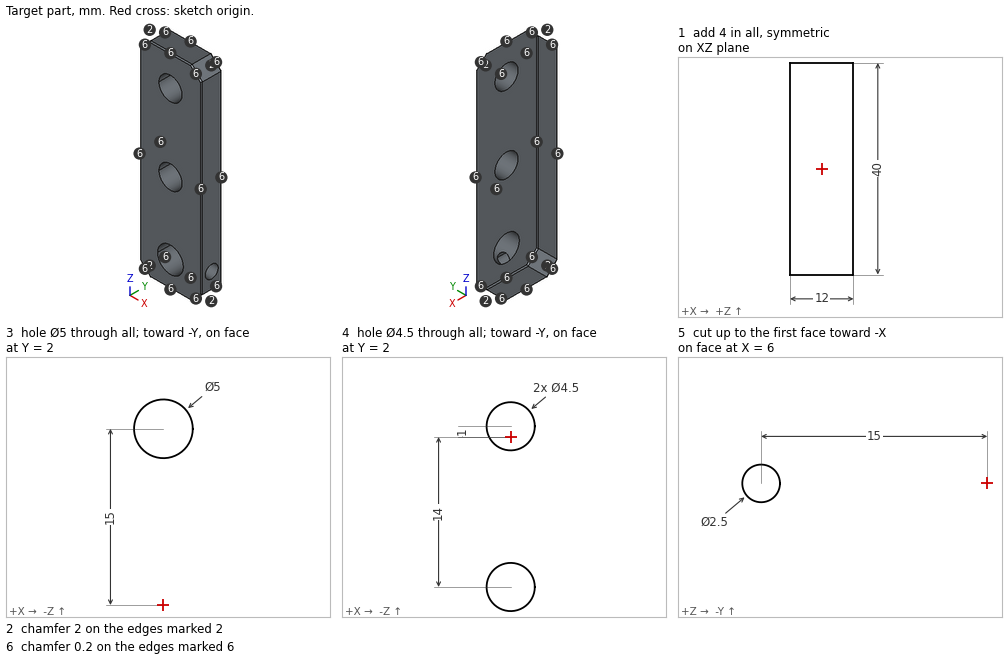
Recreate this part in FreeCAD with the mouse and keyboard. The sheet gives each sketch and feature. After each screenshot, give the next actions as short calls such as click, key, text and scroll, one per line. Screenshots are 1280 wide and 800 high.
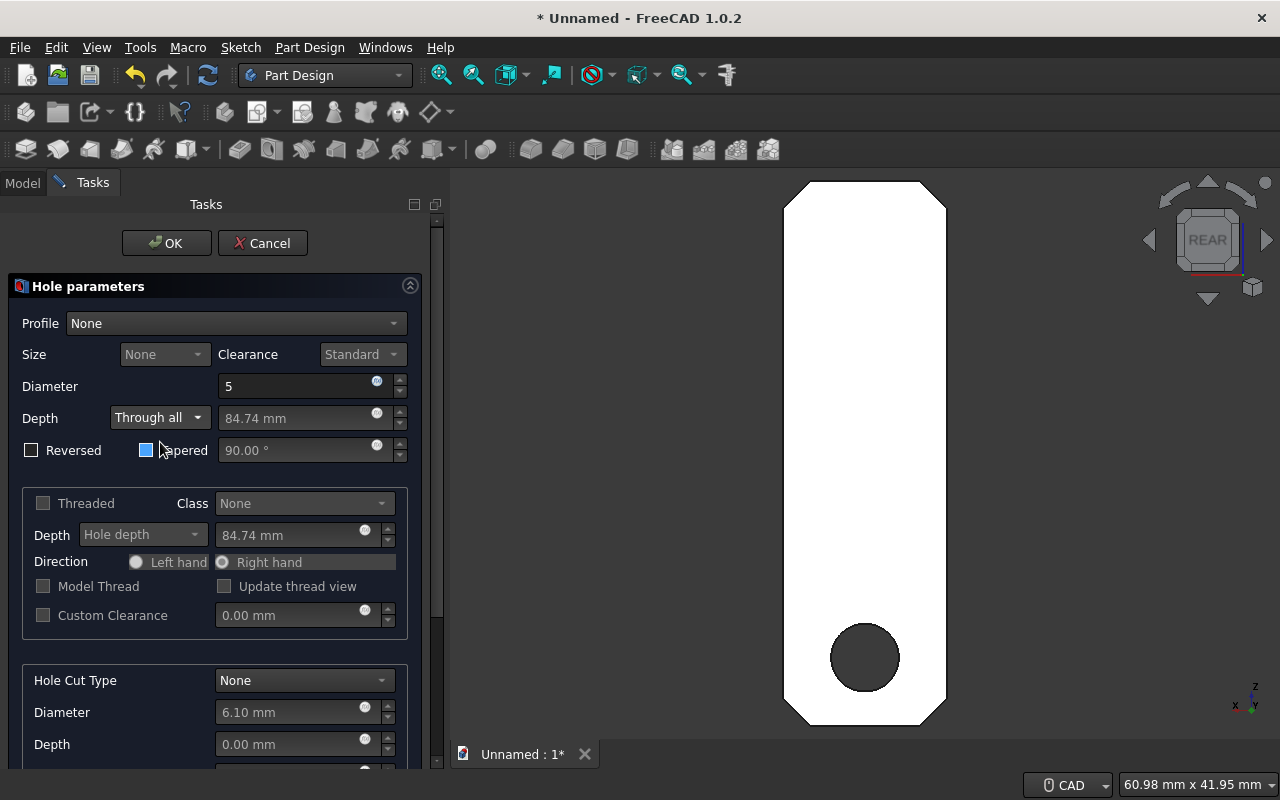
click(167, 243)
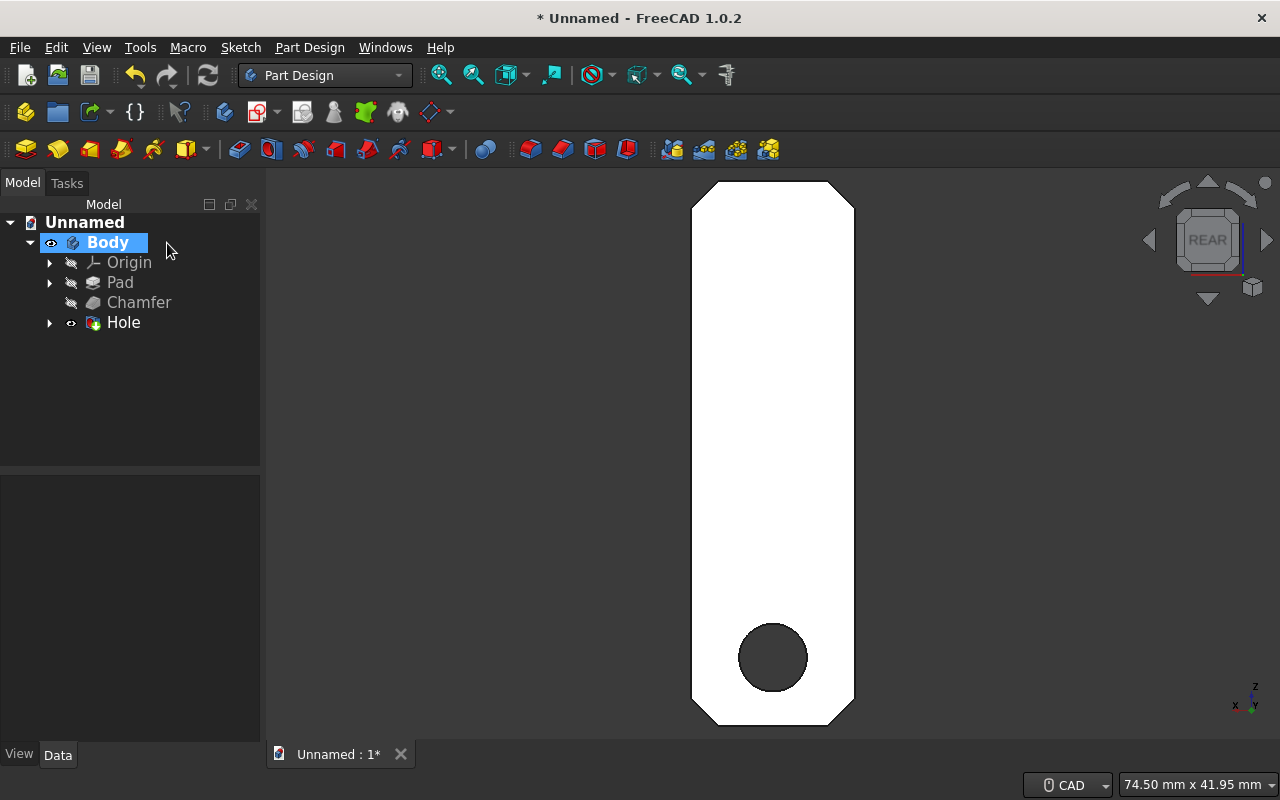
click(773, 297)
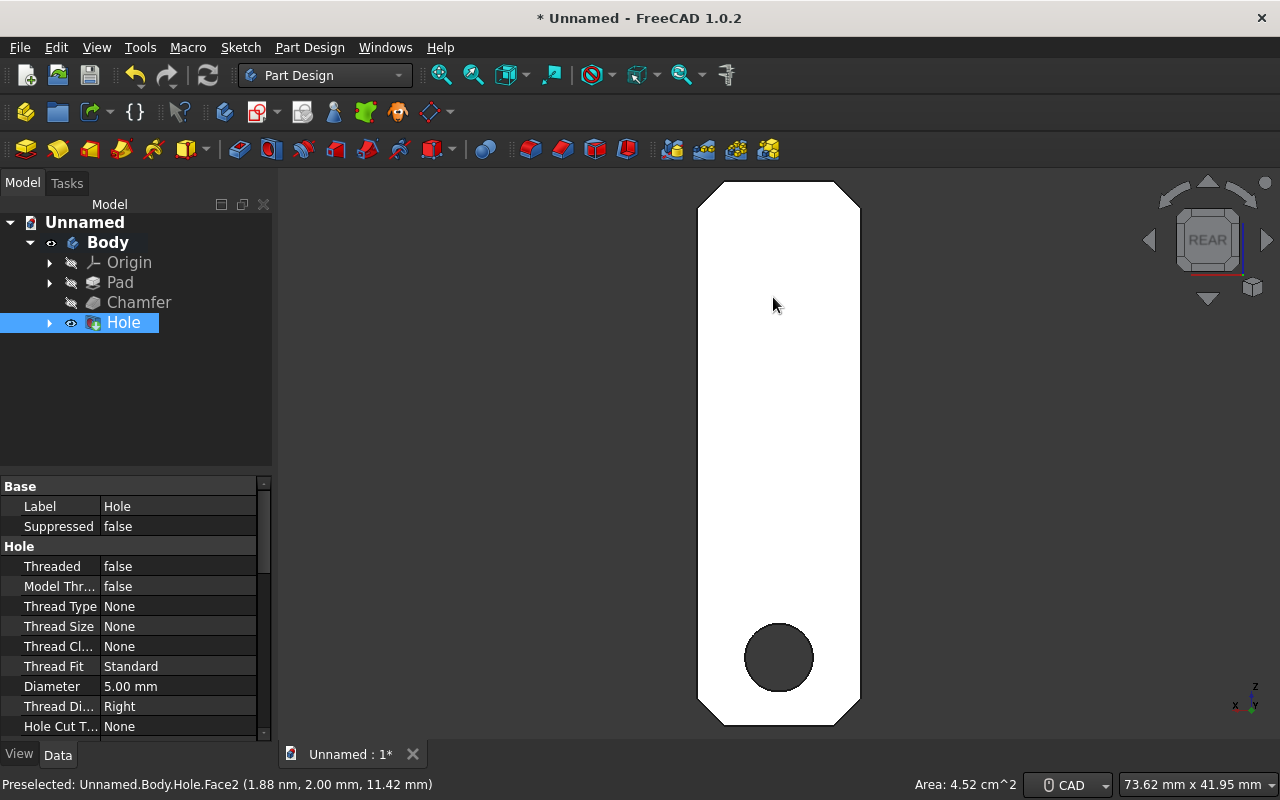
click(258, 112)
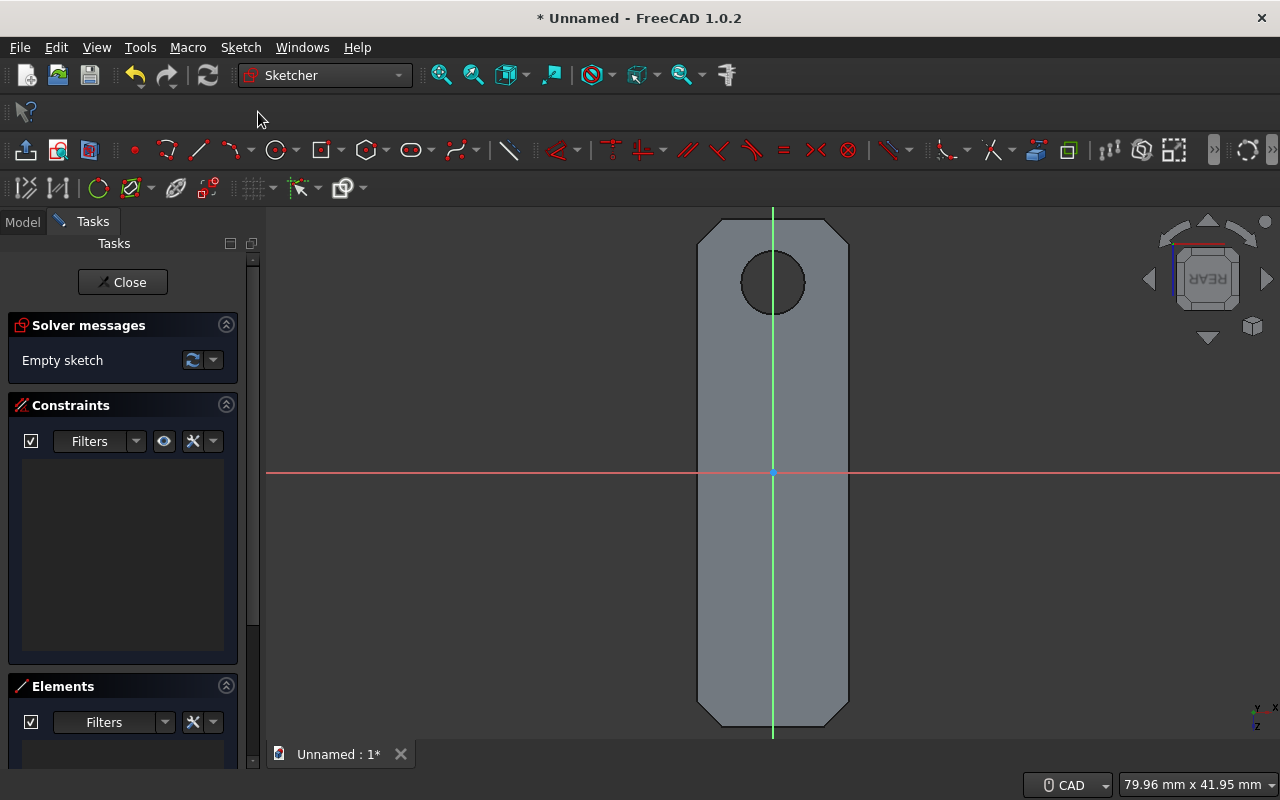
scroll(912, 711, up, 2)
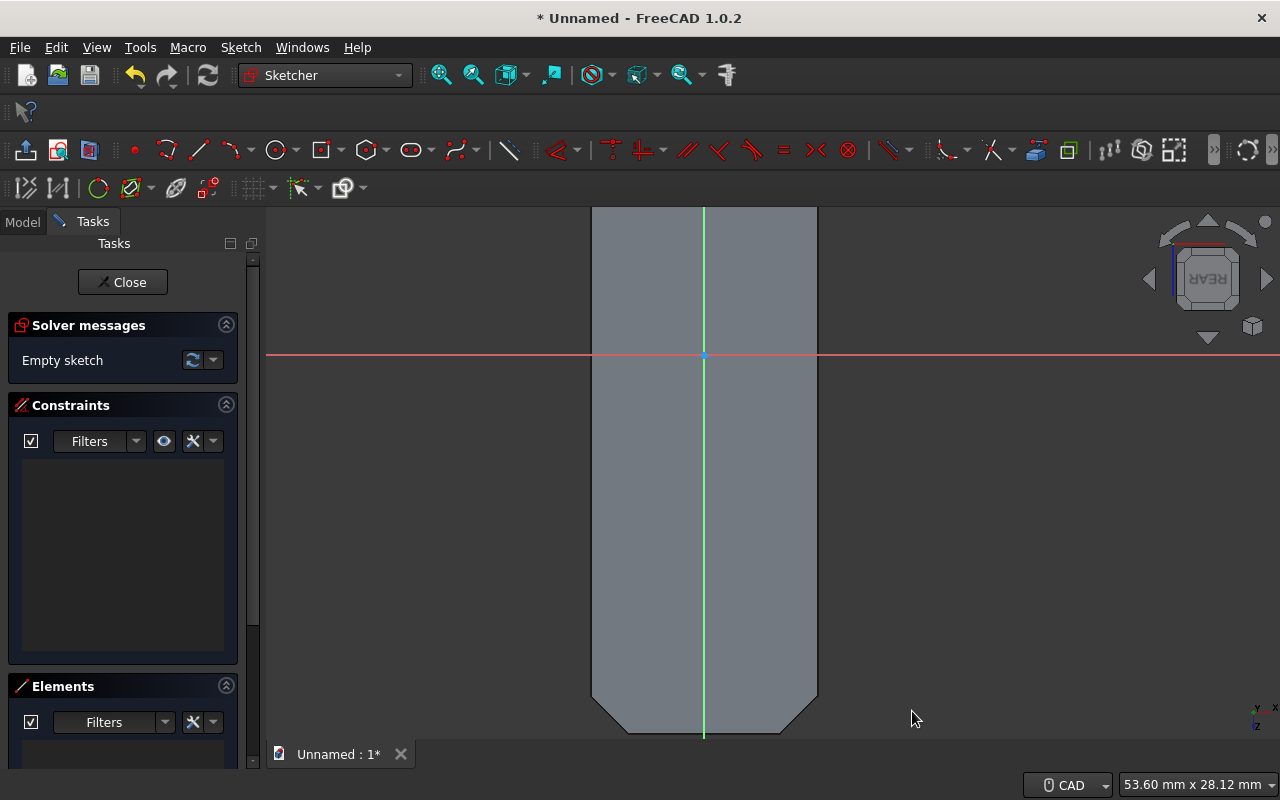
click(276, 150)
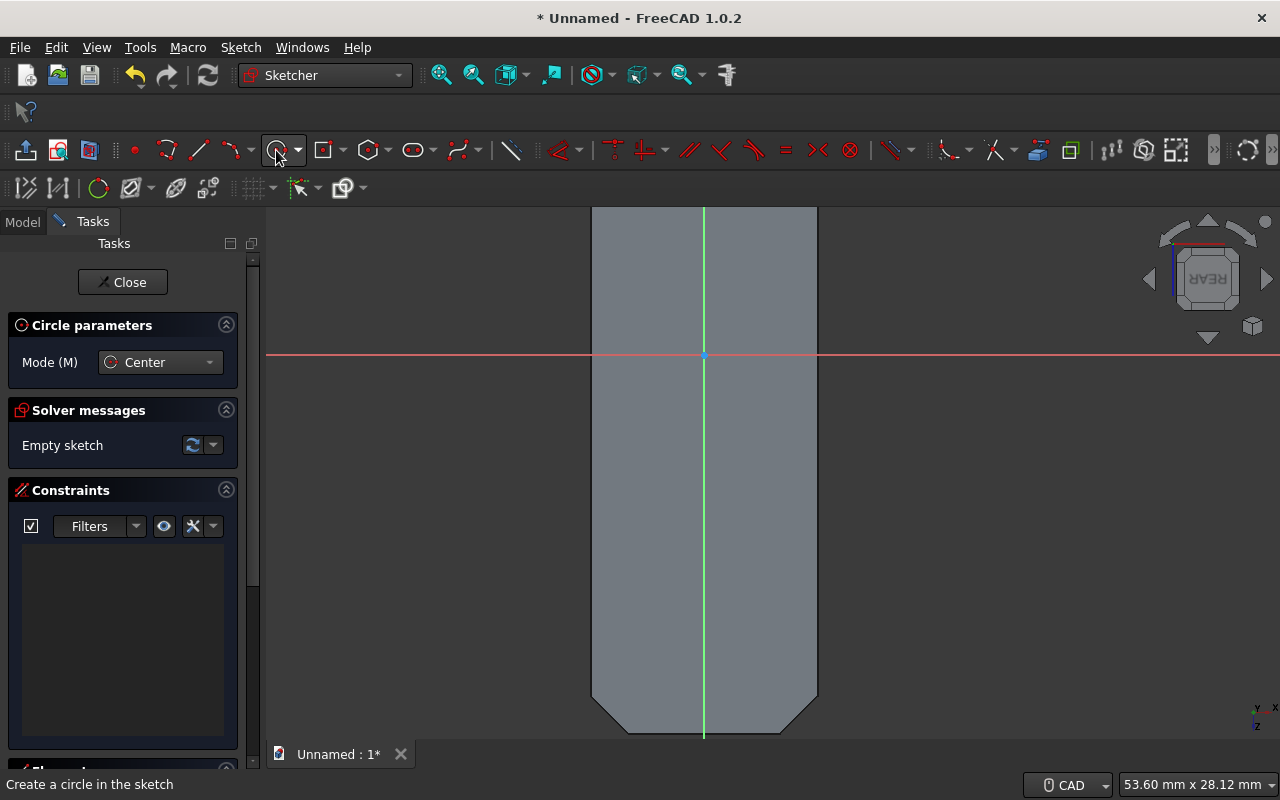
click(704, 337)
click(734, 306)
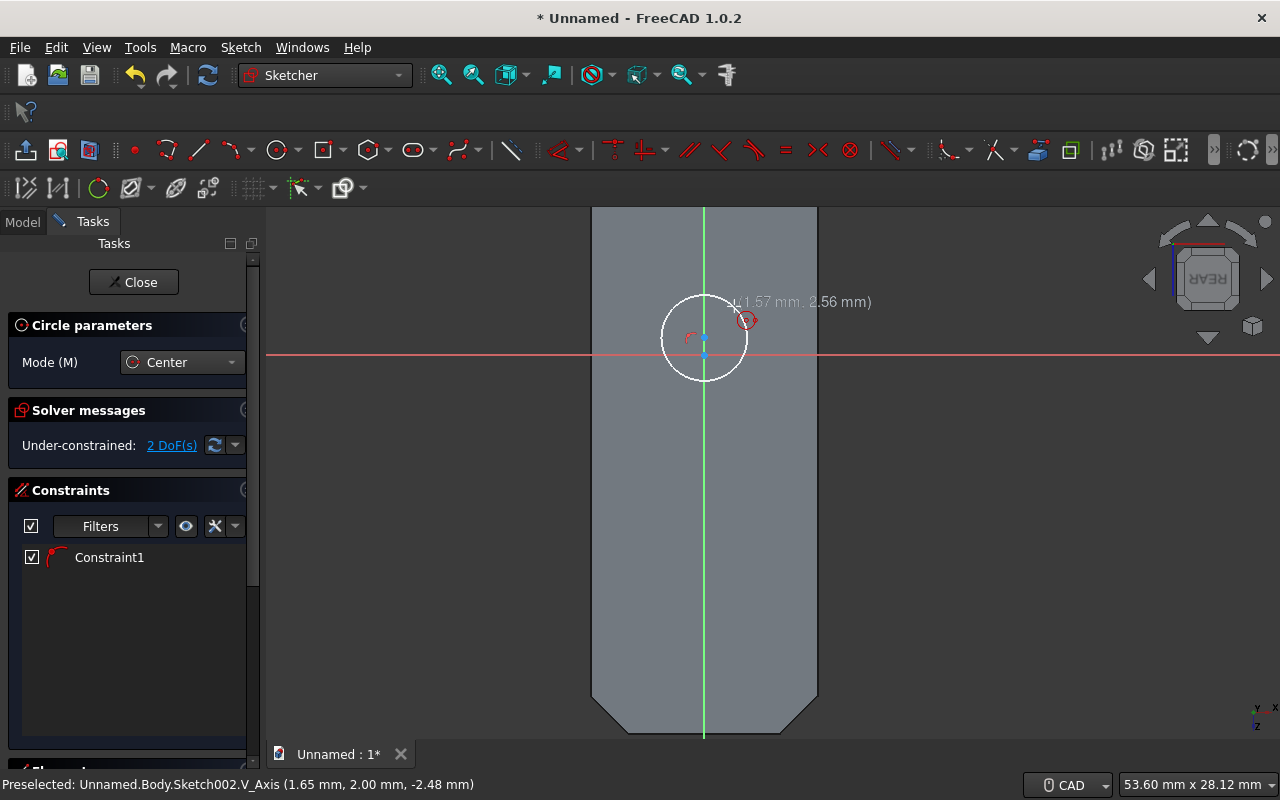
click(704, 620)
click(734, 590)
key(Escape)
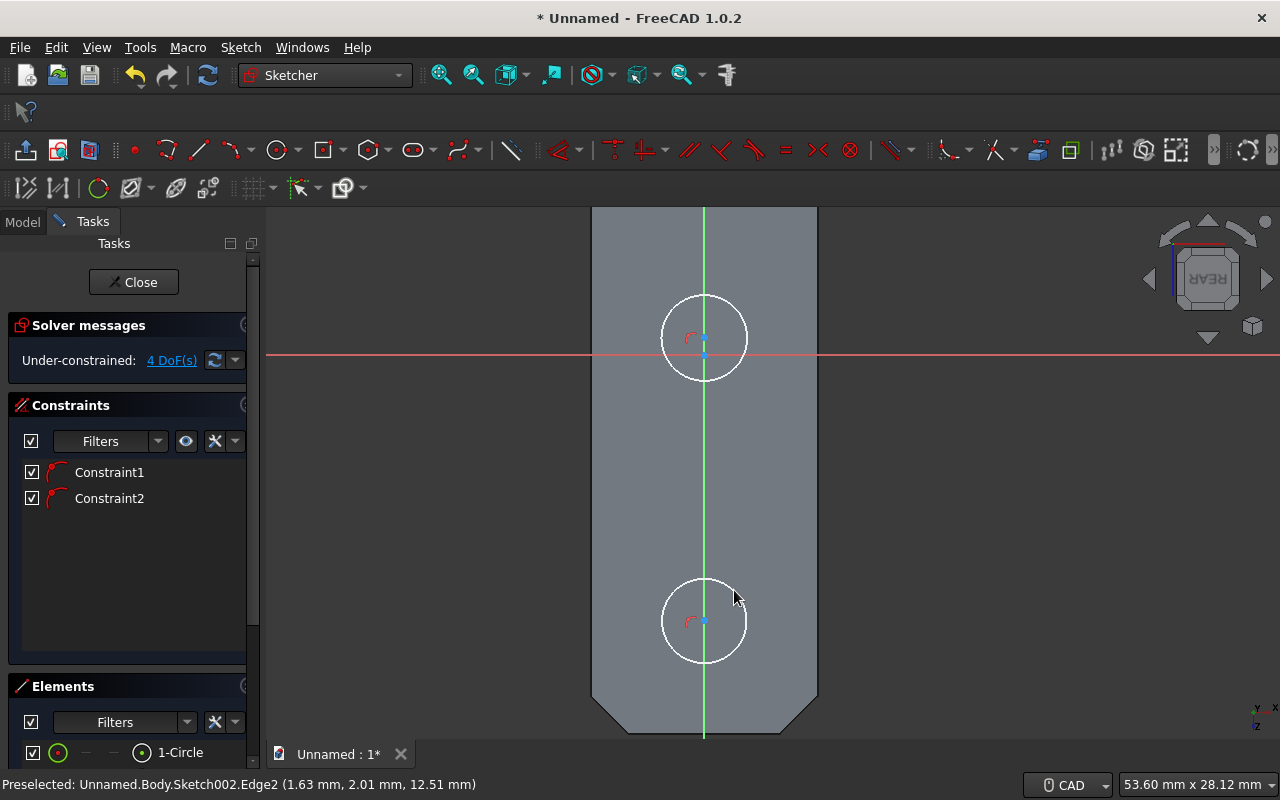
click(735, 308)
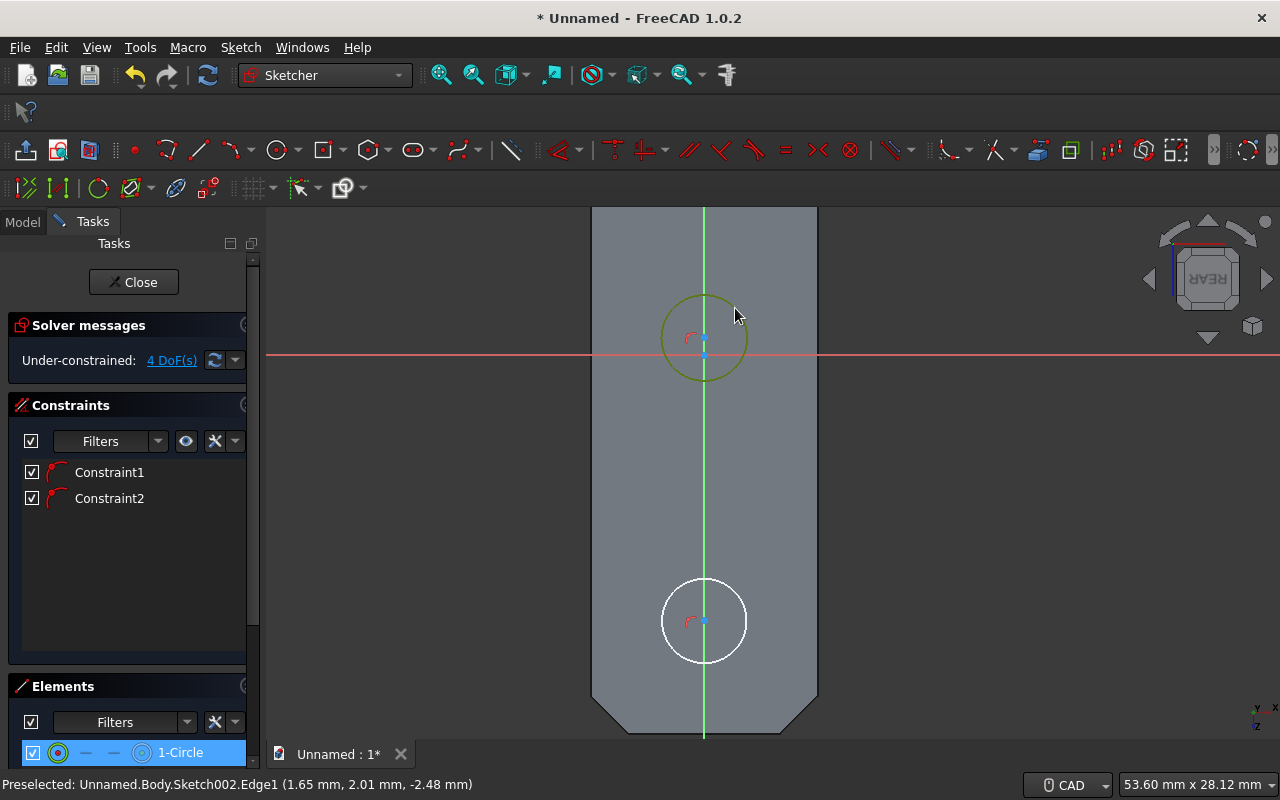
click(734, 591)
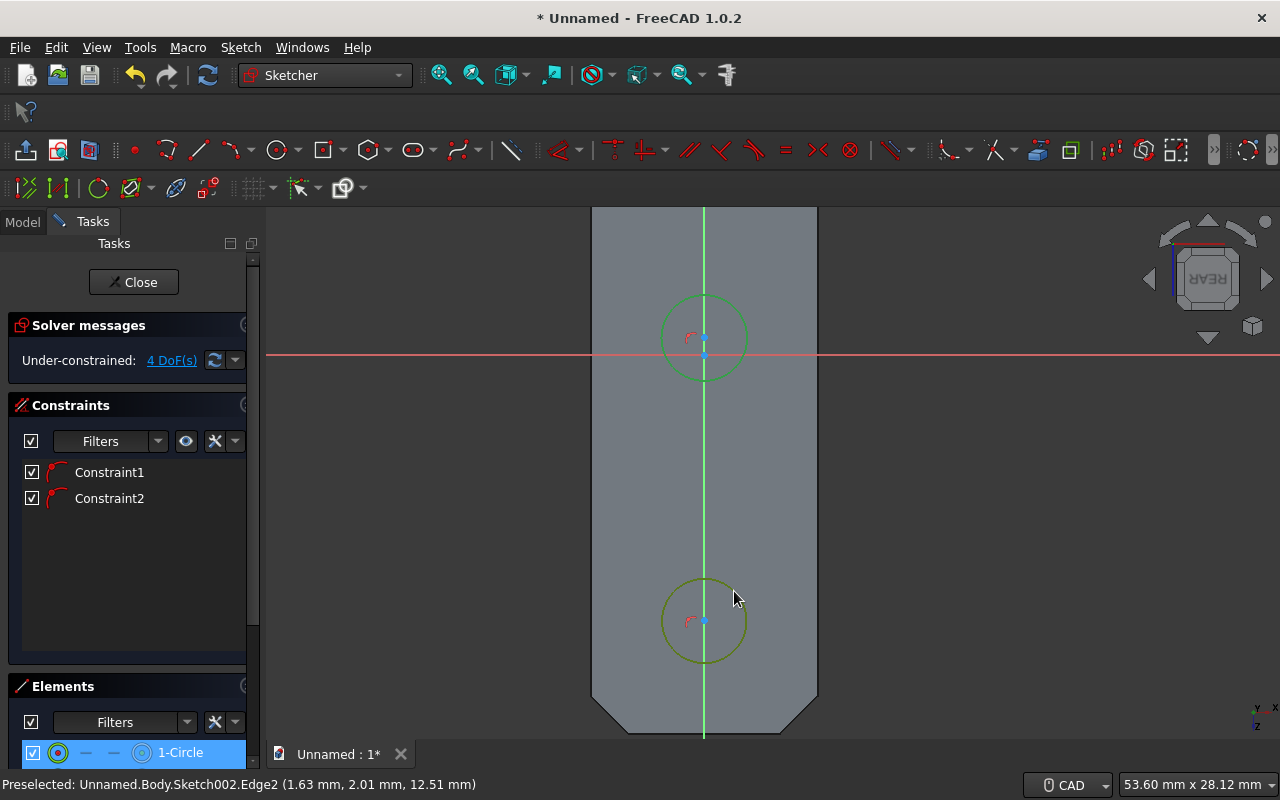
click(786, 150)